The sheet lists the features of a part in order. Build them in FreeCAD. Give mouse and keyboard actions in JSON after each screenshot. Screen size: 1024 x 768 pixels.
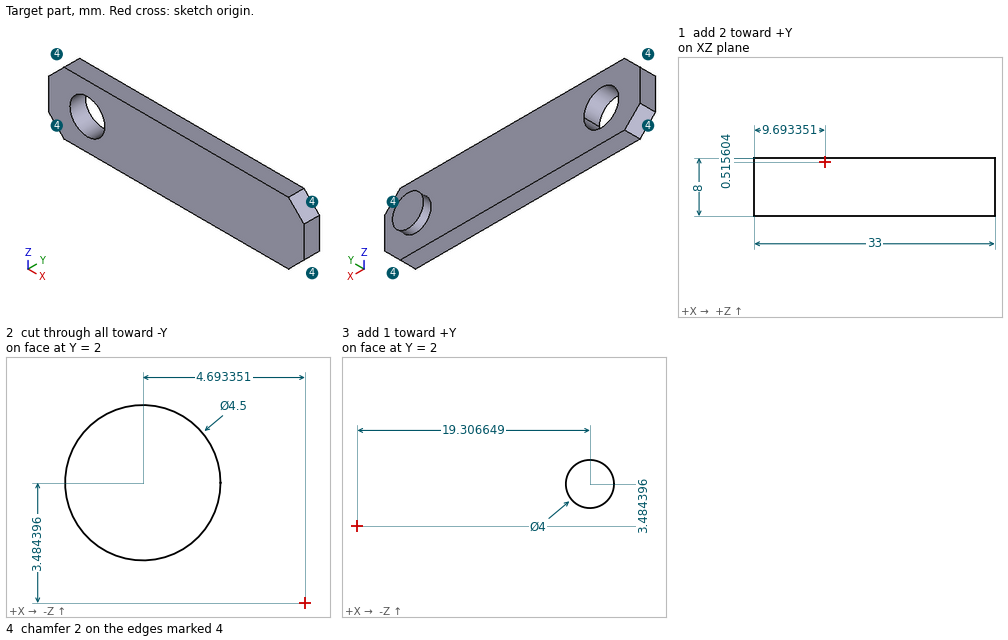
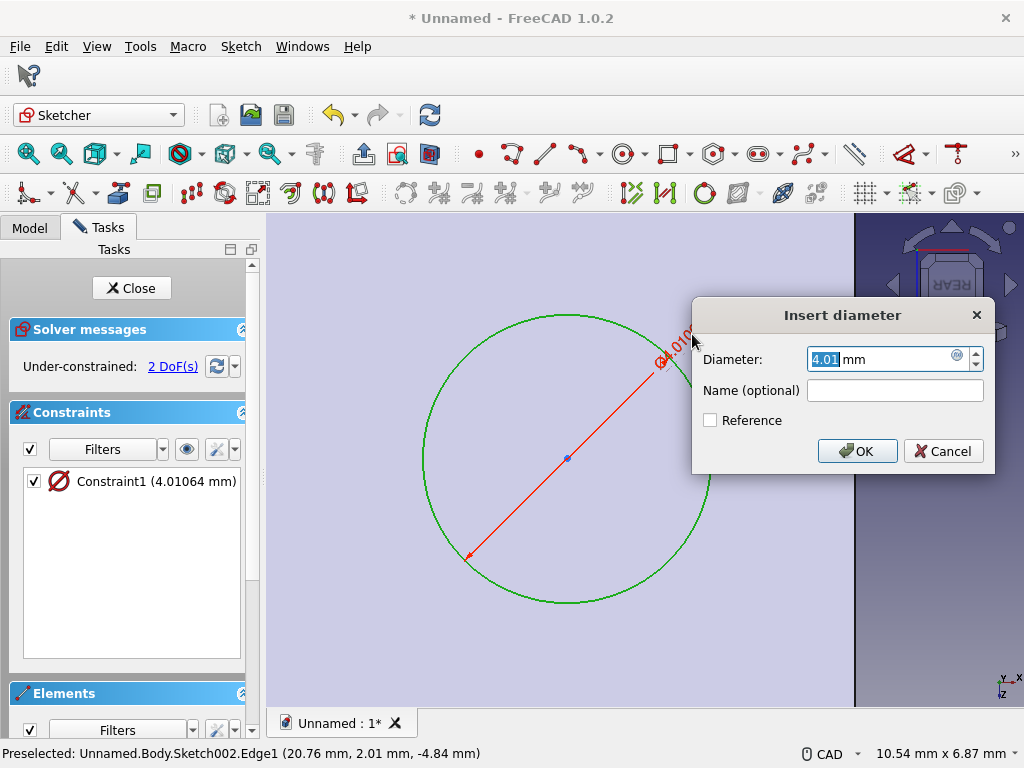
{"action": "type", "text": "4"}
{"action": "key", "text": "Return"}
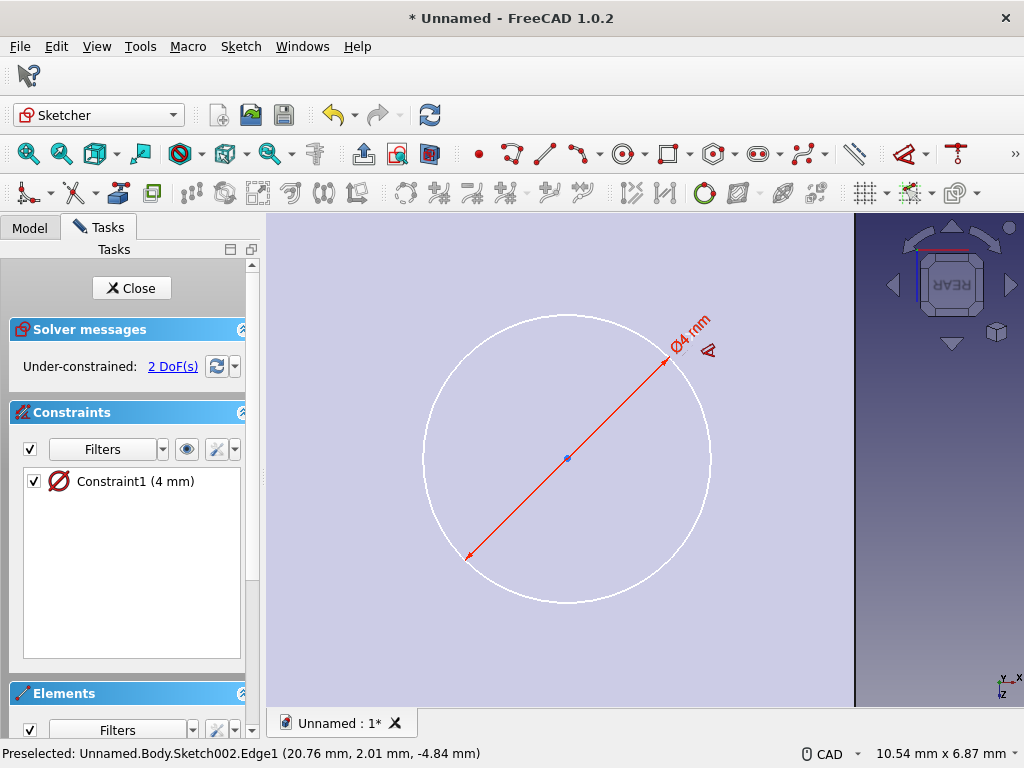
{"action": "left_click", "coordinate": [567, 459]}
{"action": "left_click", "coordinate": [601, 569]}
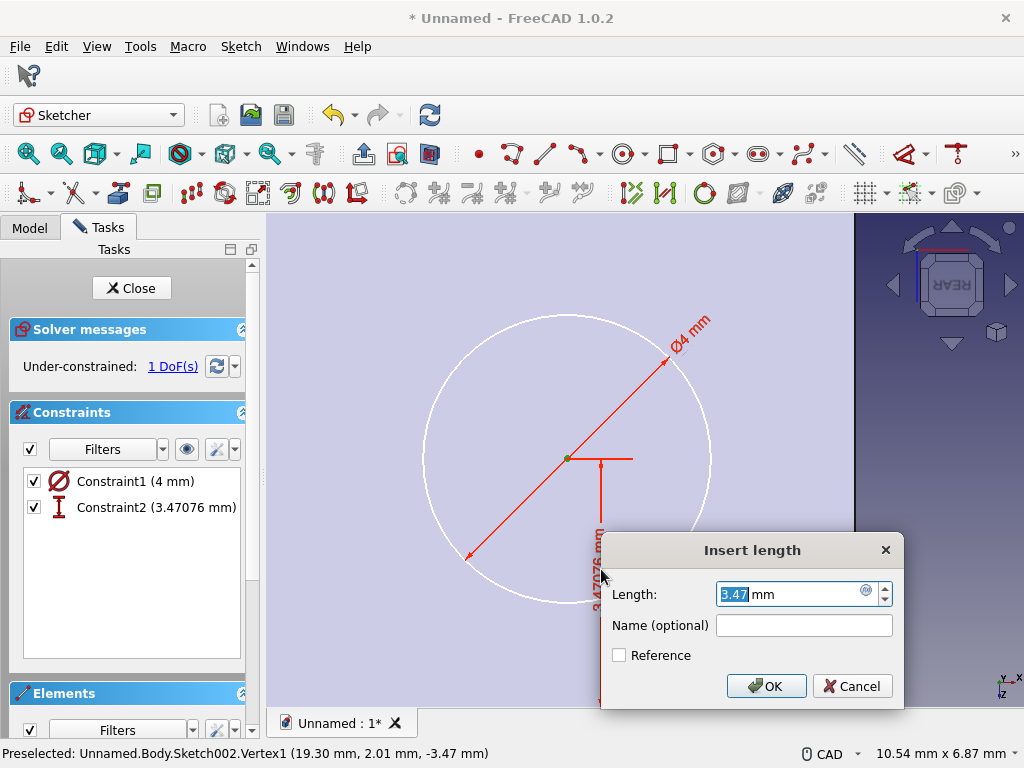
{"action": "type", "text": "3.484396"}
{"action": "key", "text": "Return"}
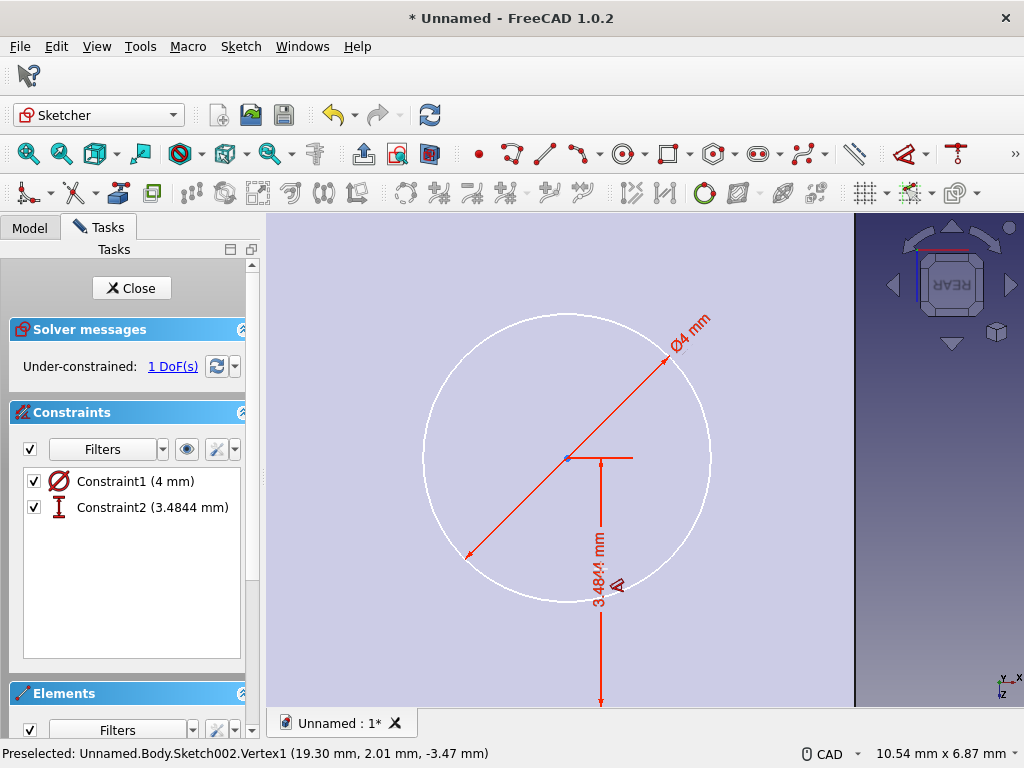
{"action": "left_click", "coordinate": [567, 458]}
{"action": "left_click", "coordinate": [368, 424]}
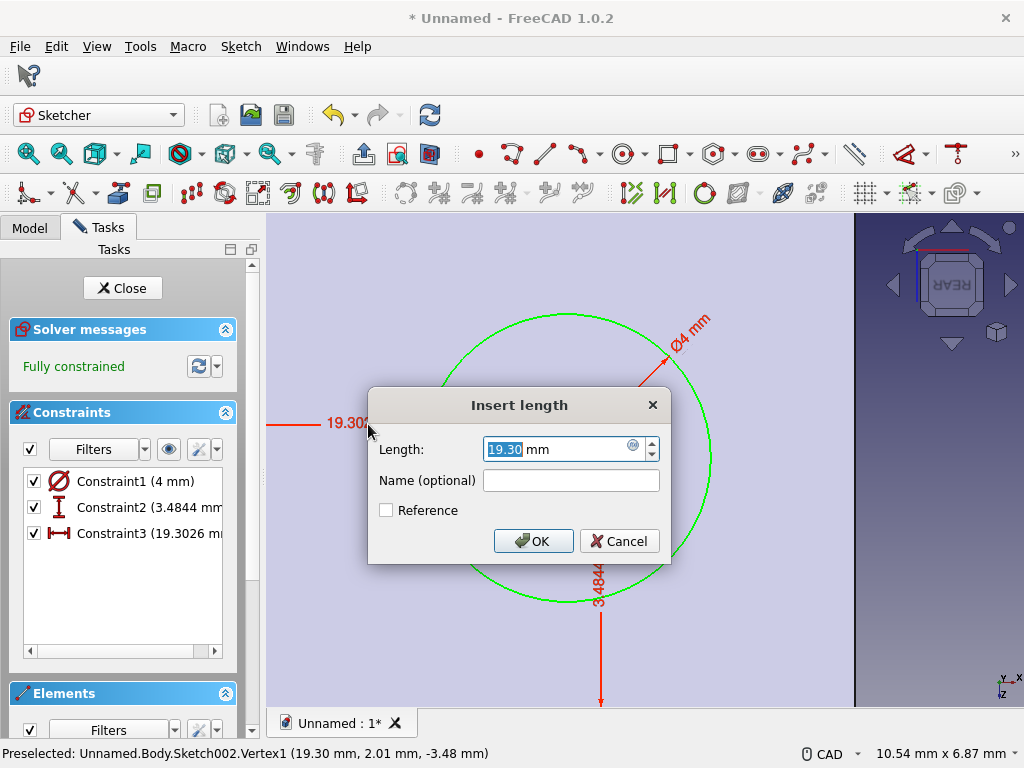
{"action": "type", "text": "19.306649"}
{"action": "key", "text": "Return"}
{"action": "key", "text": "Escape"}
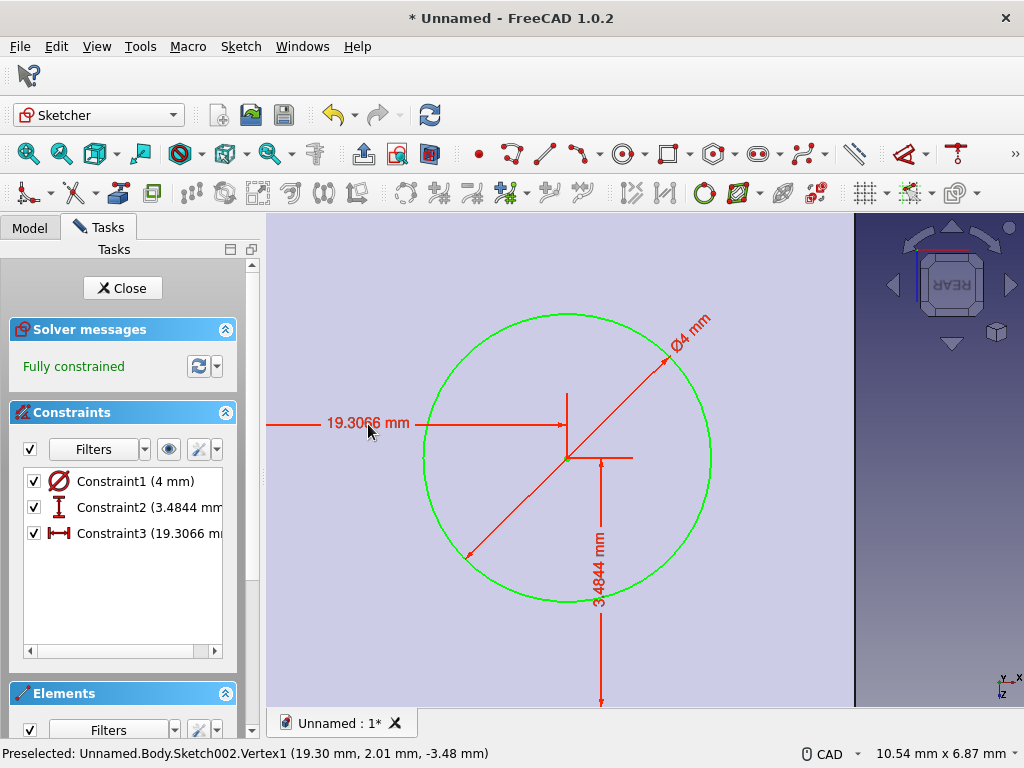
{"action": "left_click", "coordinate": [123, 288]}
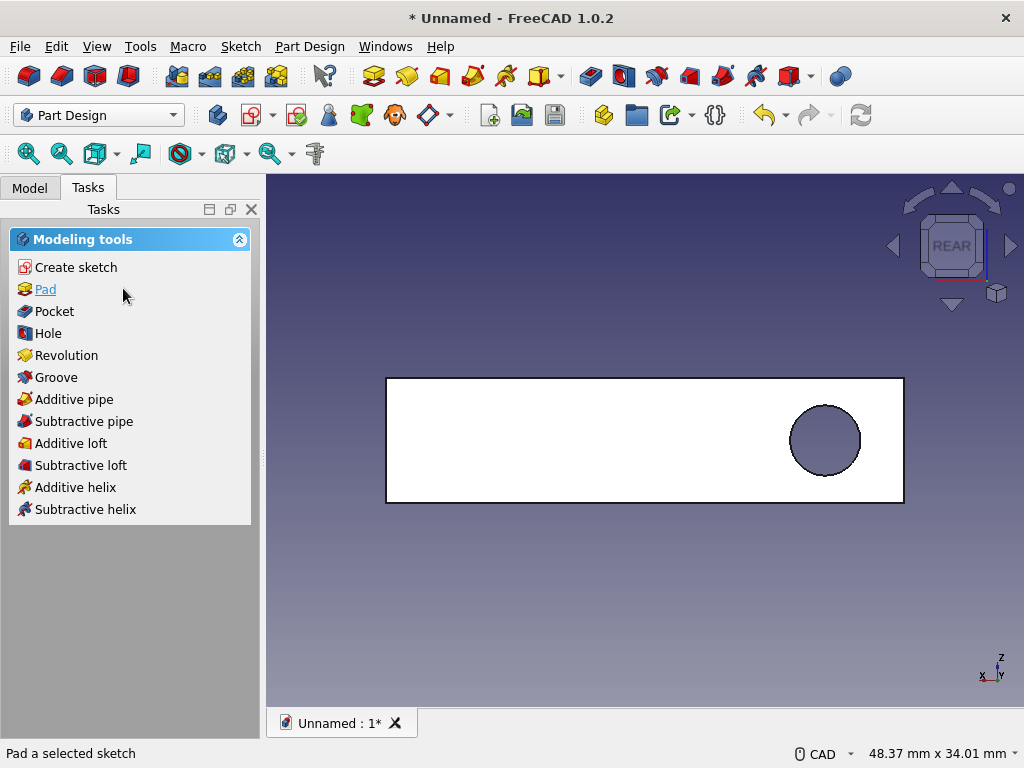
{"action": "left_click", "coordinate": [374, 76]}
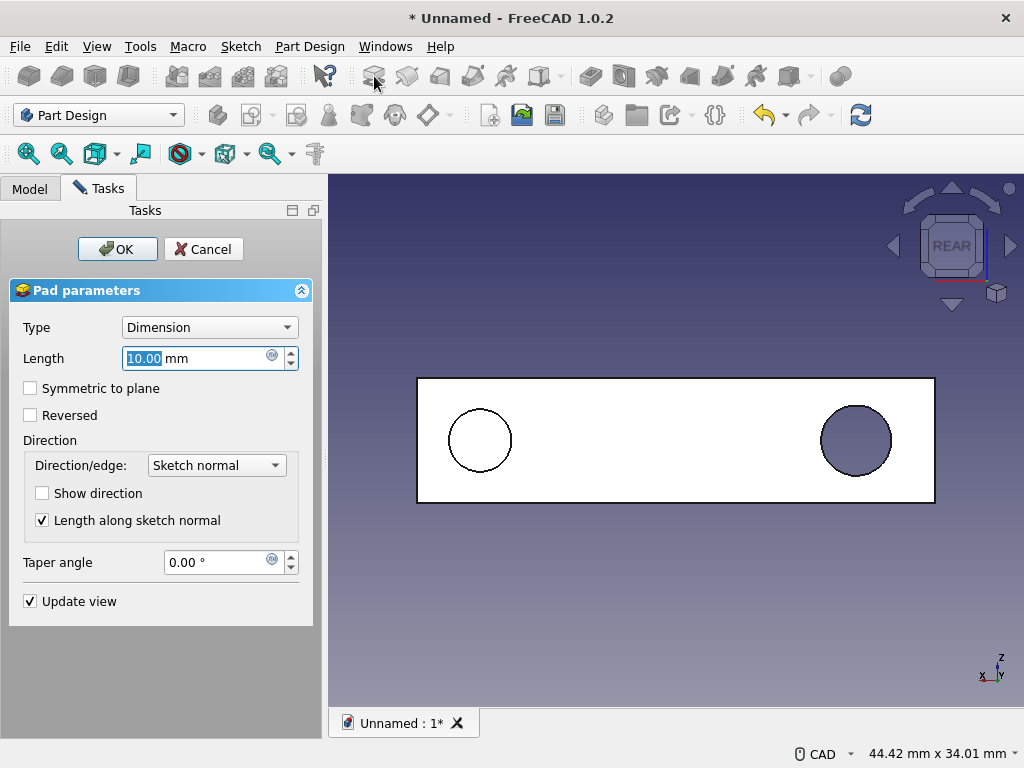
{"action": "type", "text": "1"}
{"action": "key", "text": "Tab"}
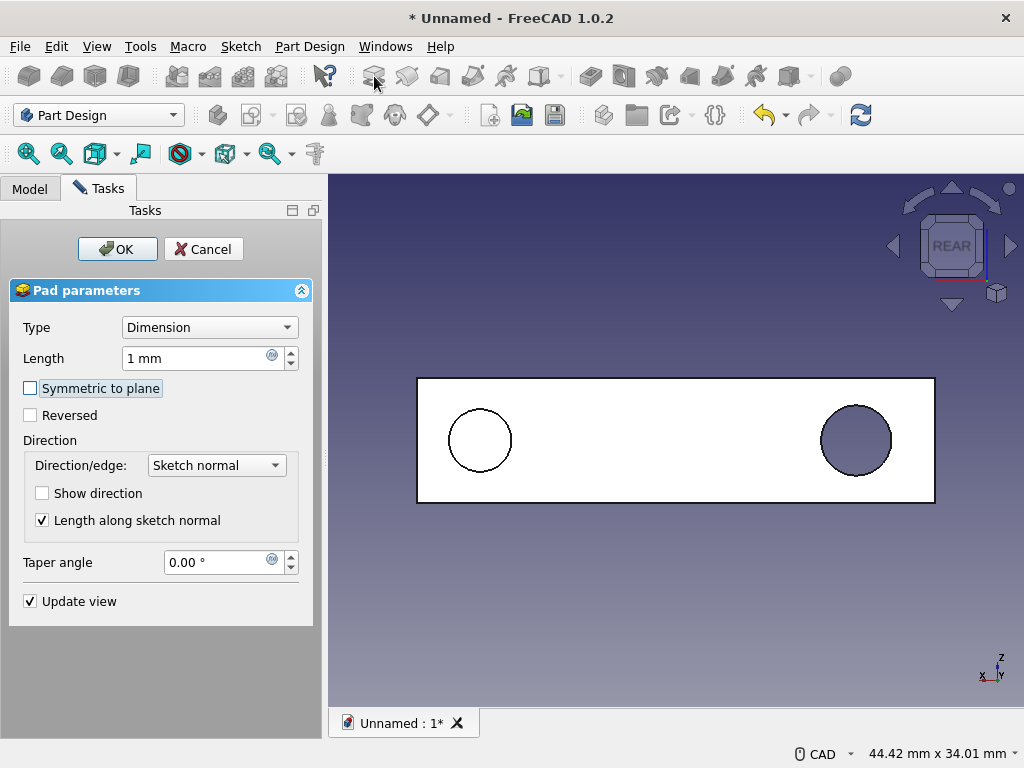
{"action": "left_click", "coordinate": [118, 249]}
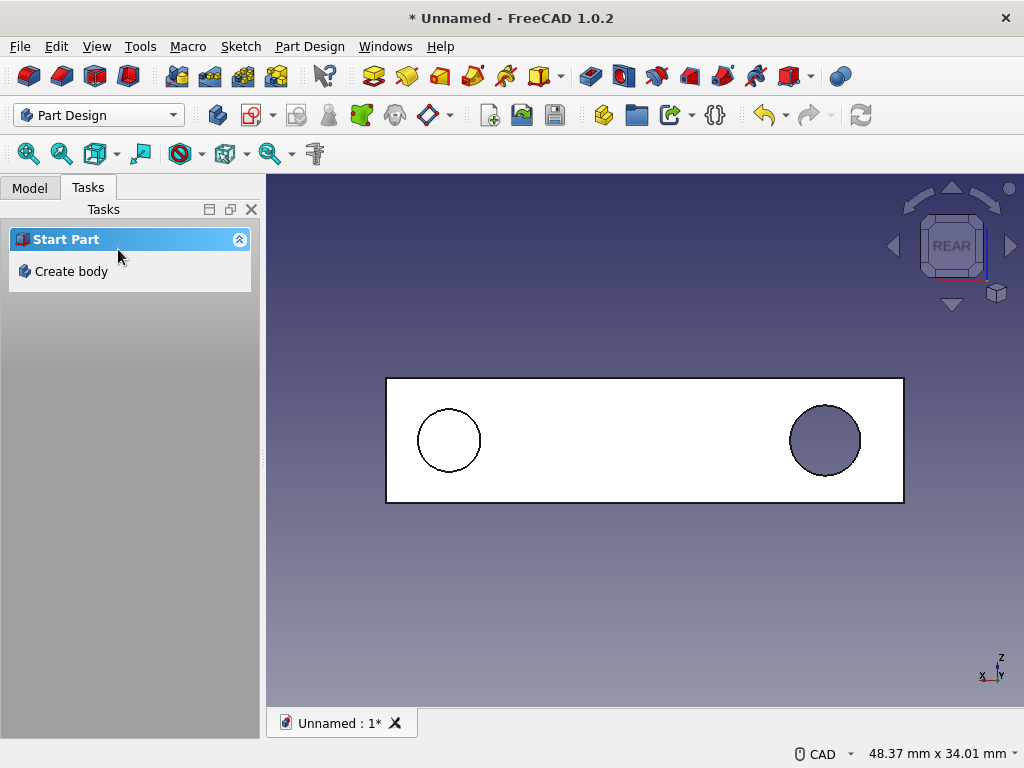
{"action": "key", "text": "0"}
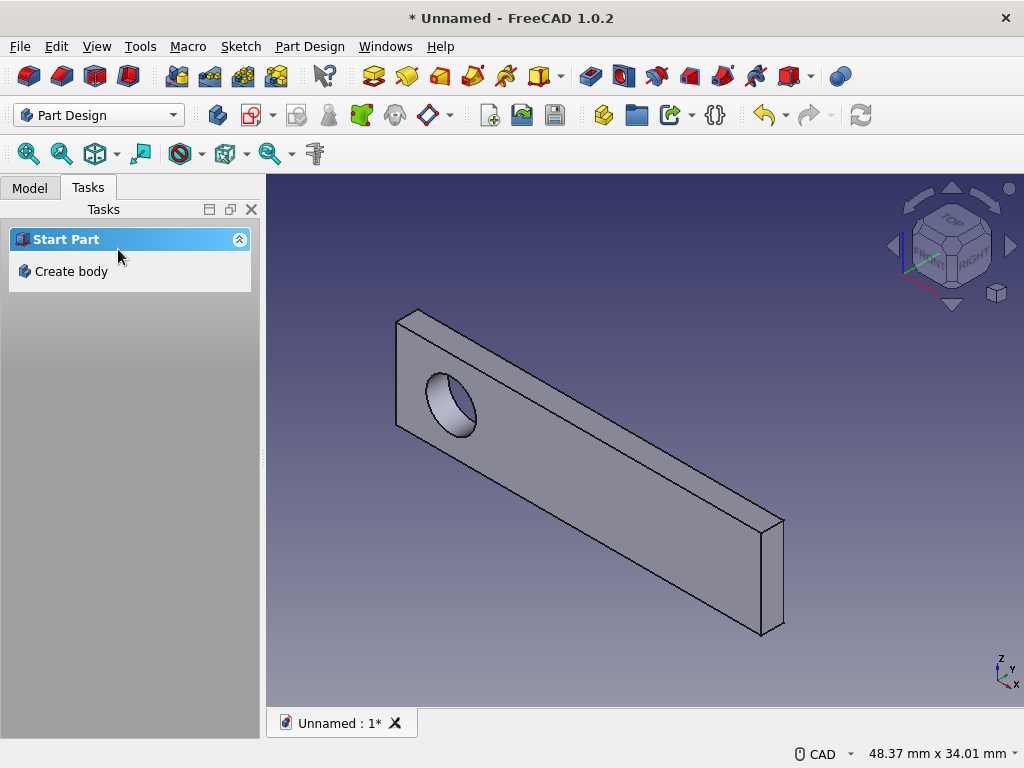
{"action": "left_click", "coordinate": [772, 526]}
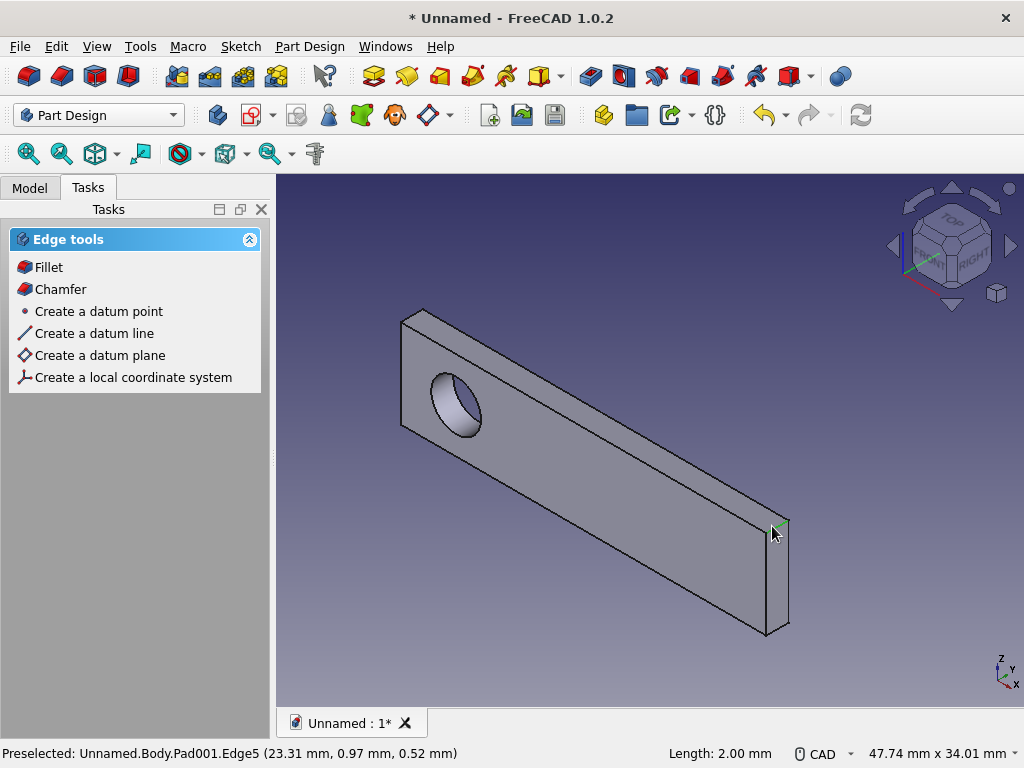
{"action": "key", "text": "2"}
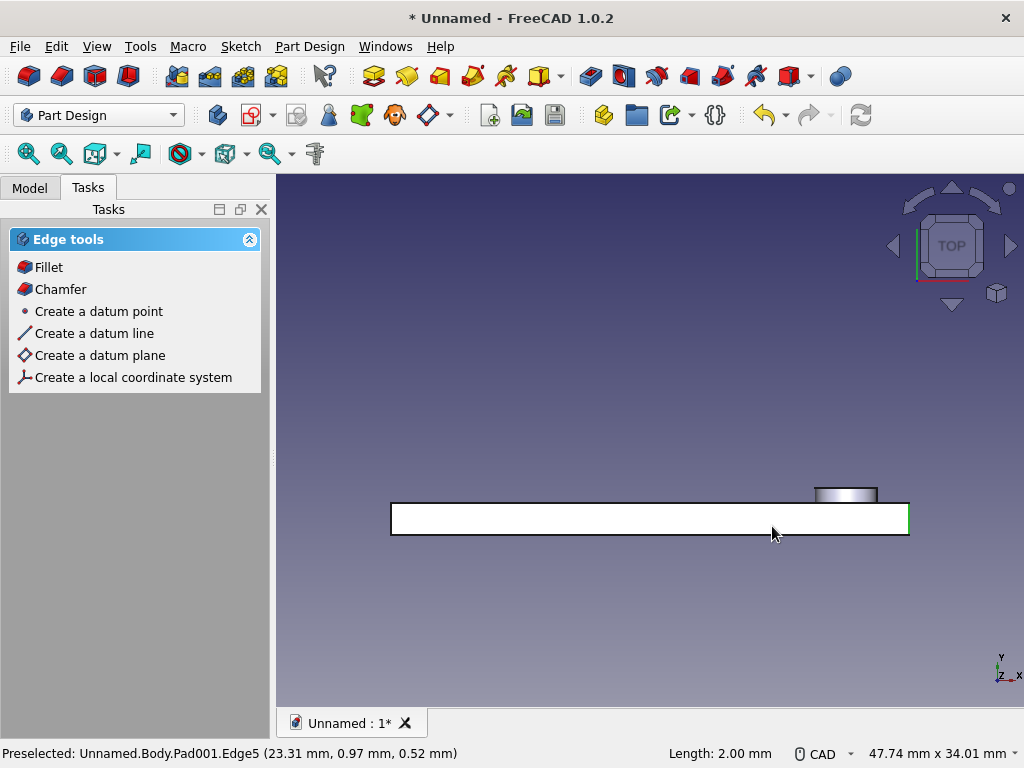
{"action": "left_click", "coordinate": [391, 518], "text": "ctrl"}